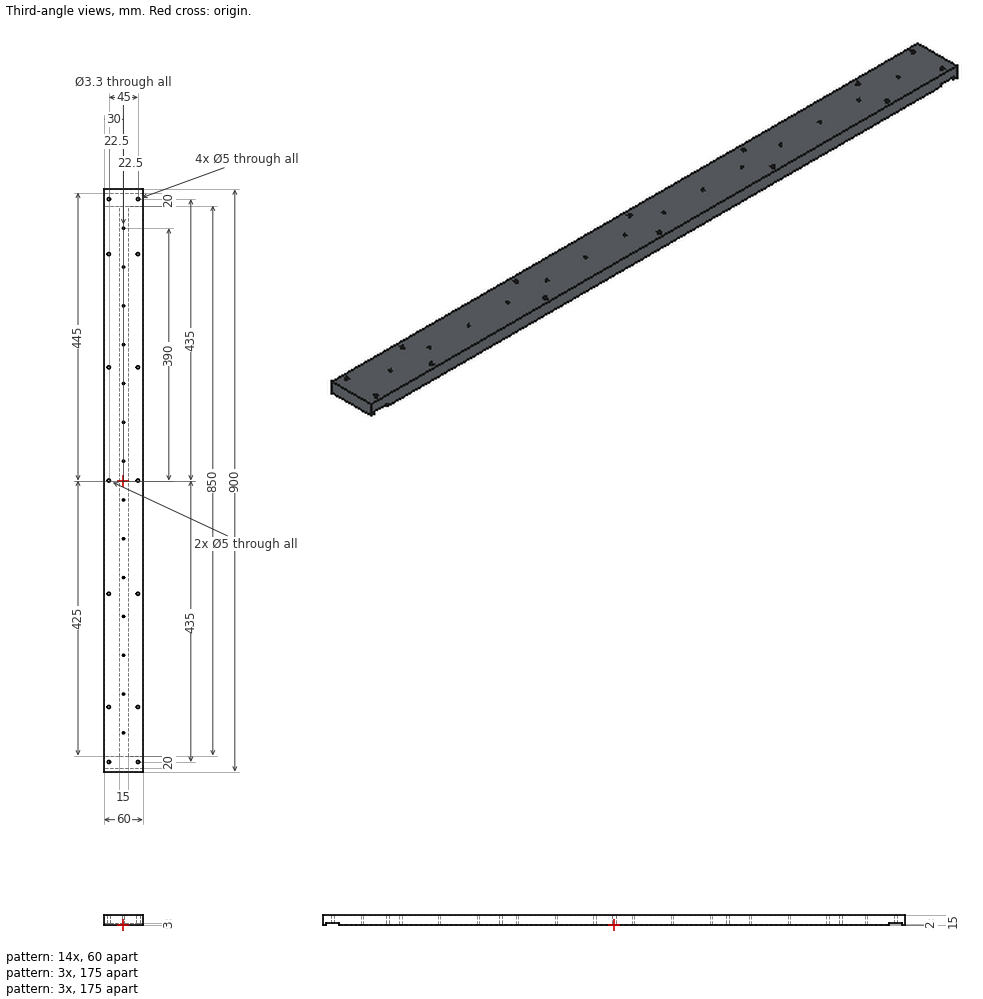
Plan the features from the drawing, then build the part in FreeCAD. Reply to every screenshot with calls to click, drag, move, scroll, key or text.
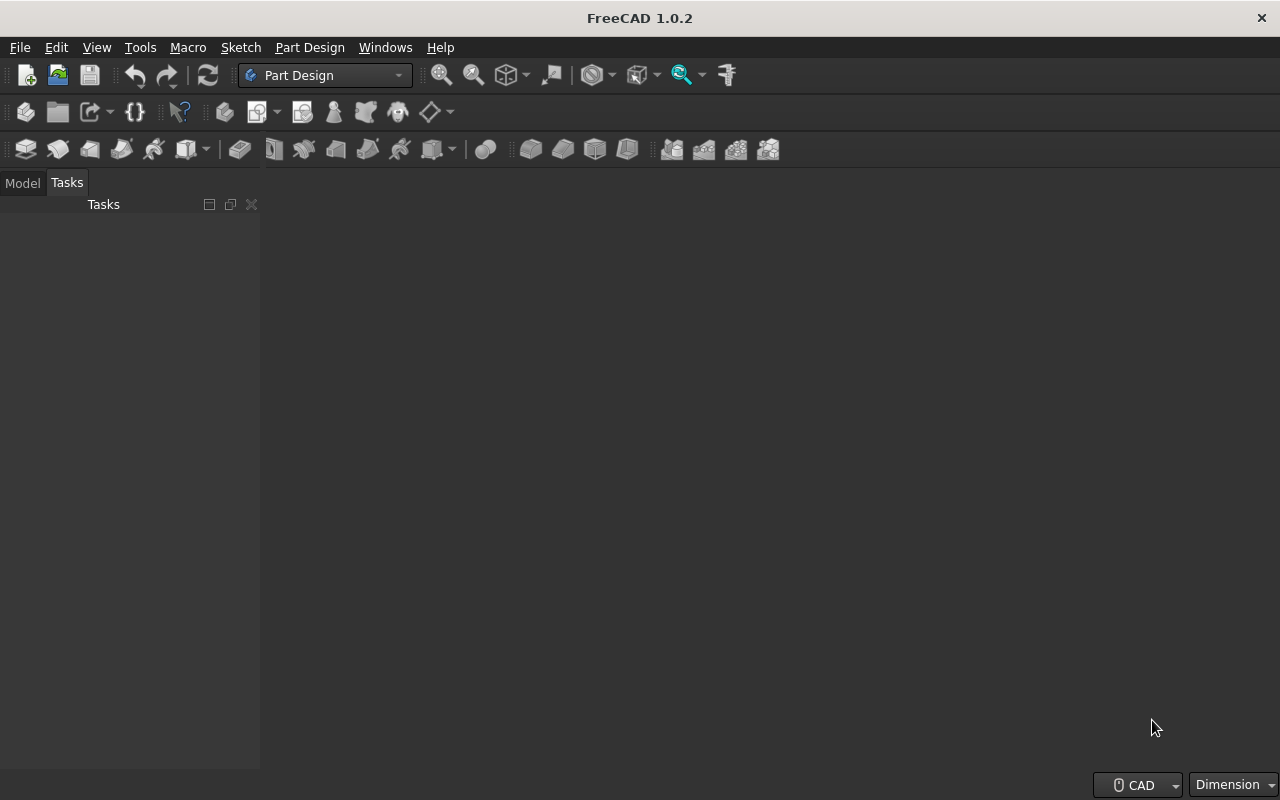
key(ctrl+n)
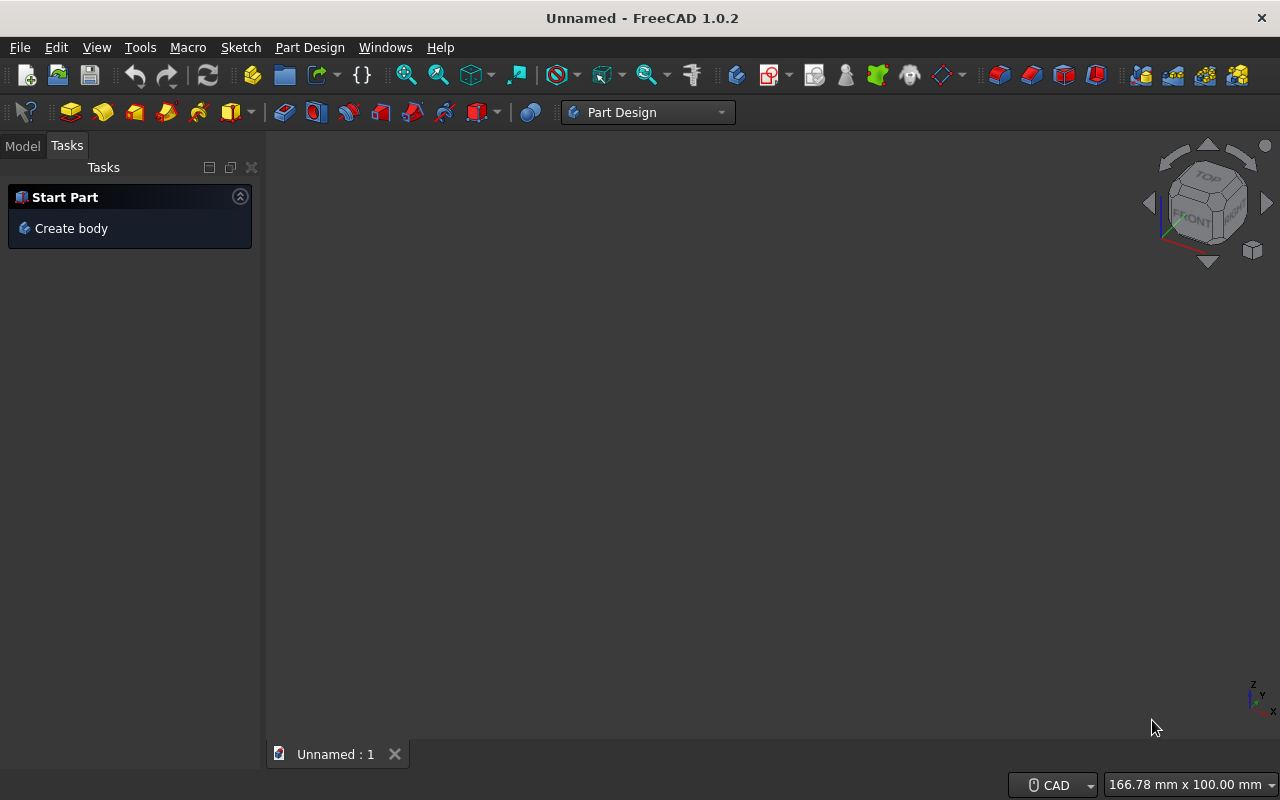
click(770, 76)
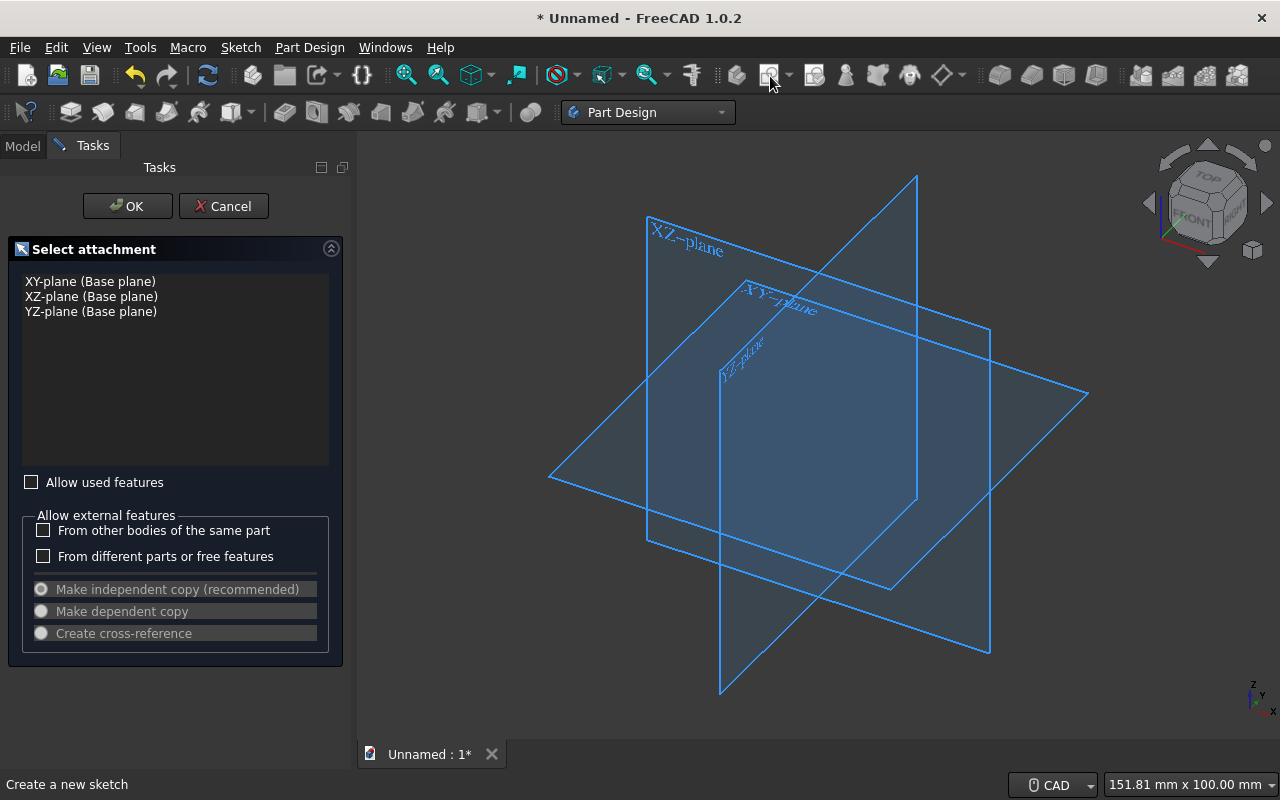
click(82, 282)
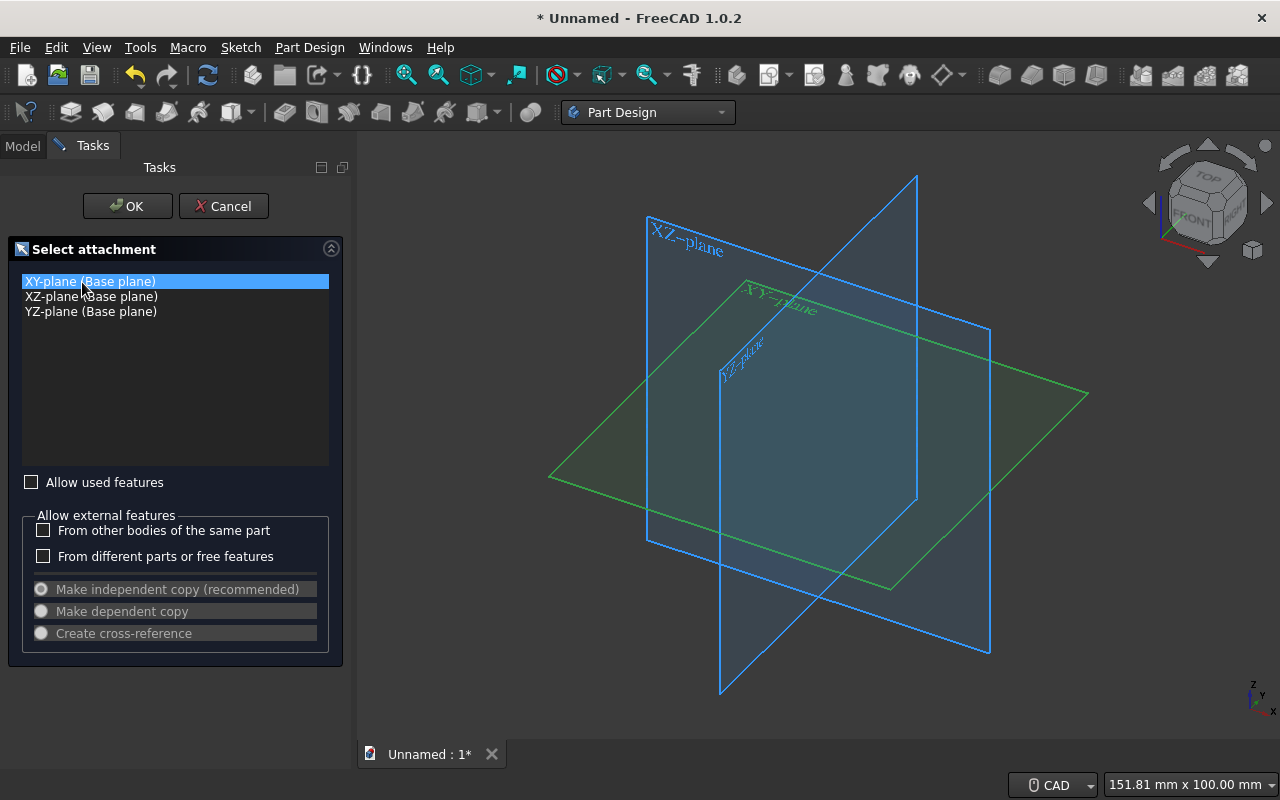
click(128, 206)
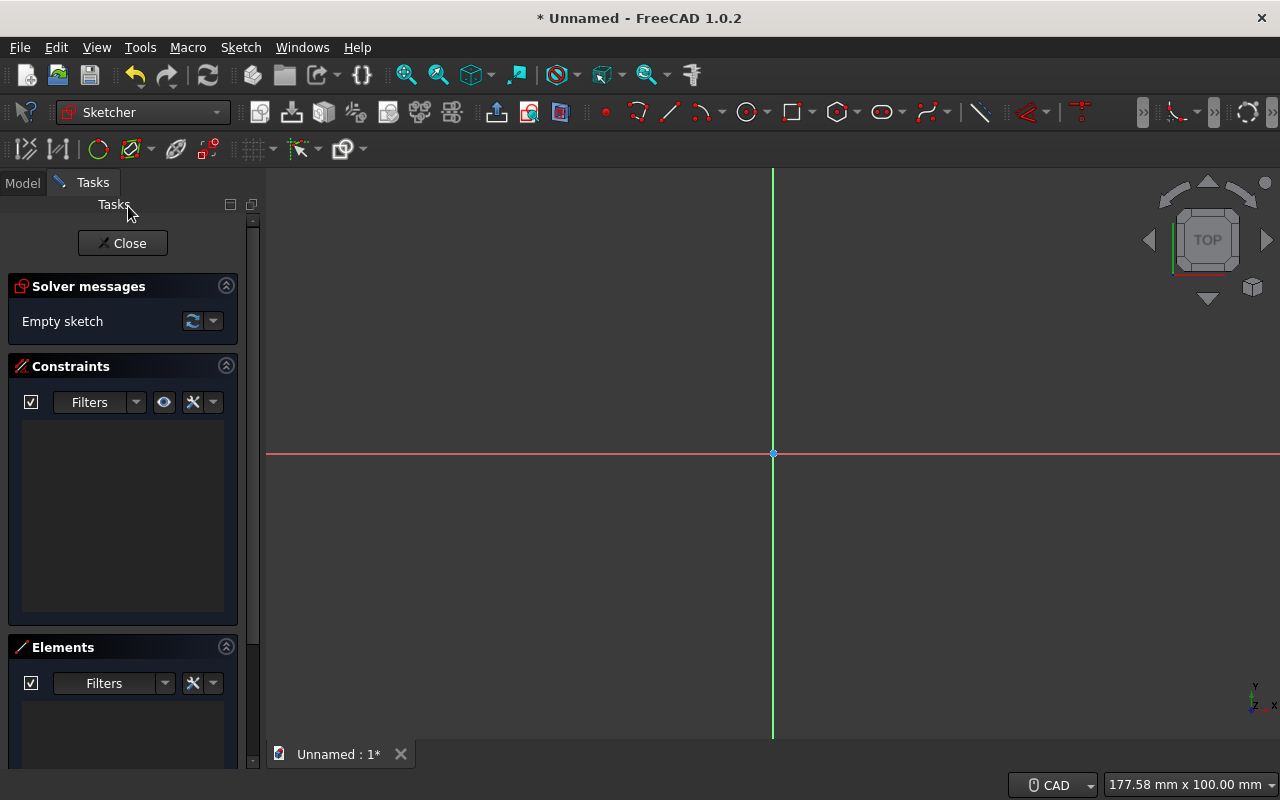
scroll(699, 454, down, 13)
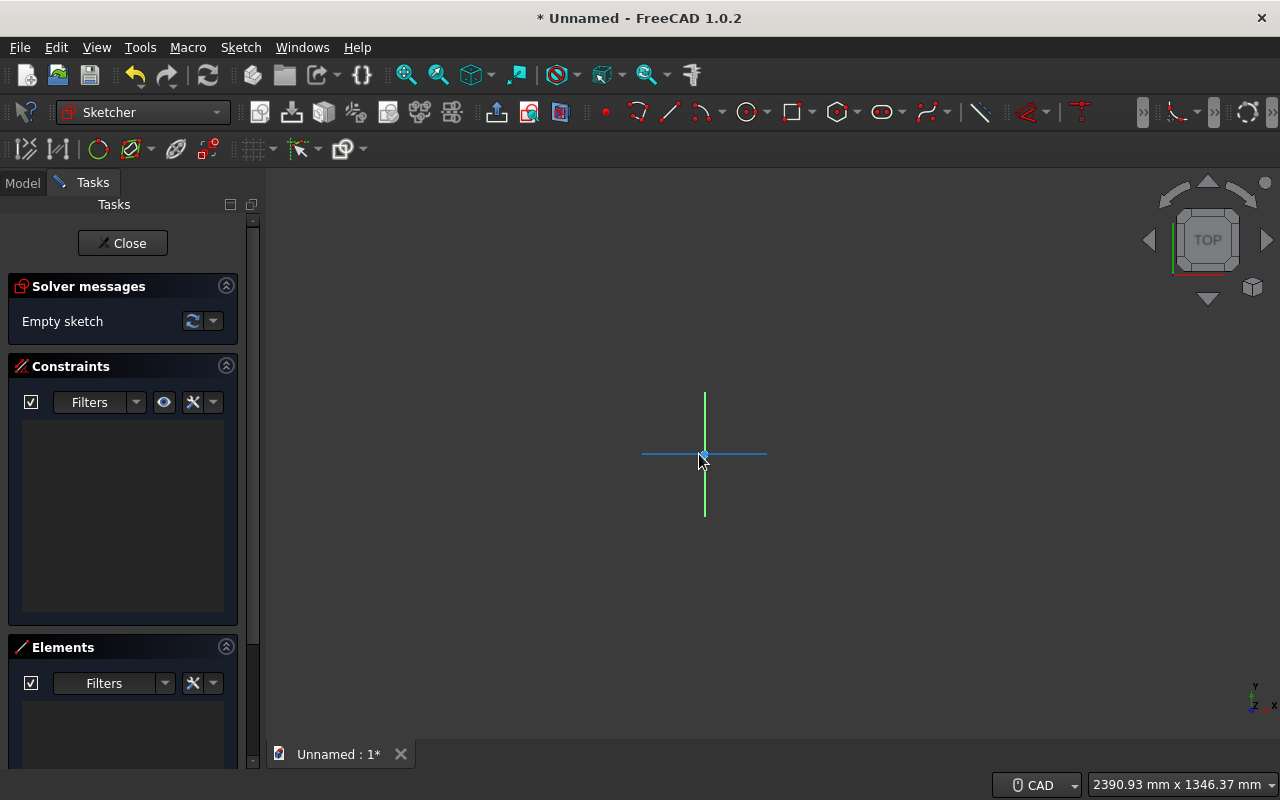
key(g)
key(v)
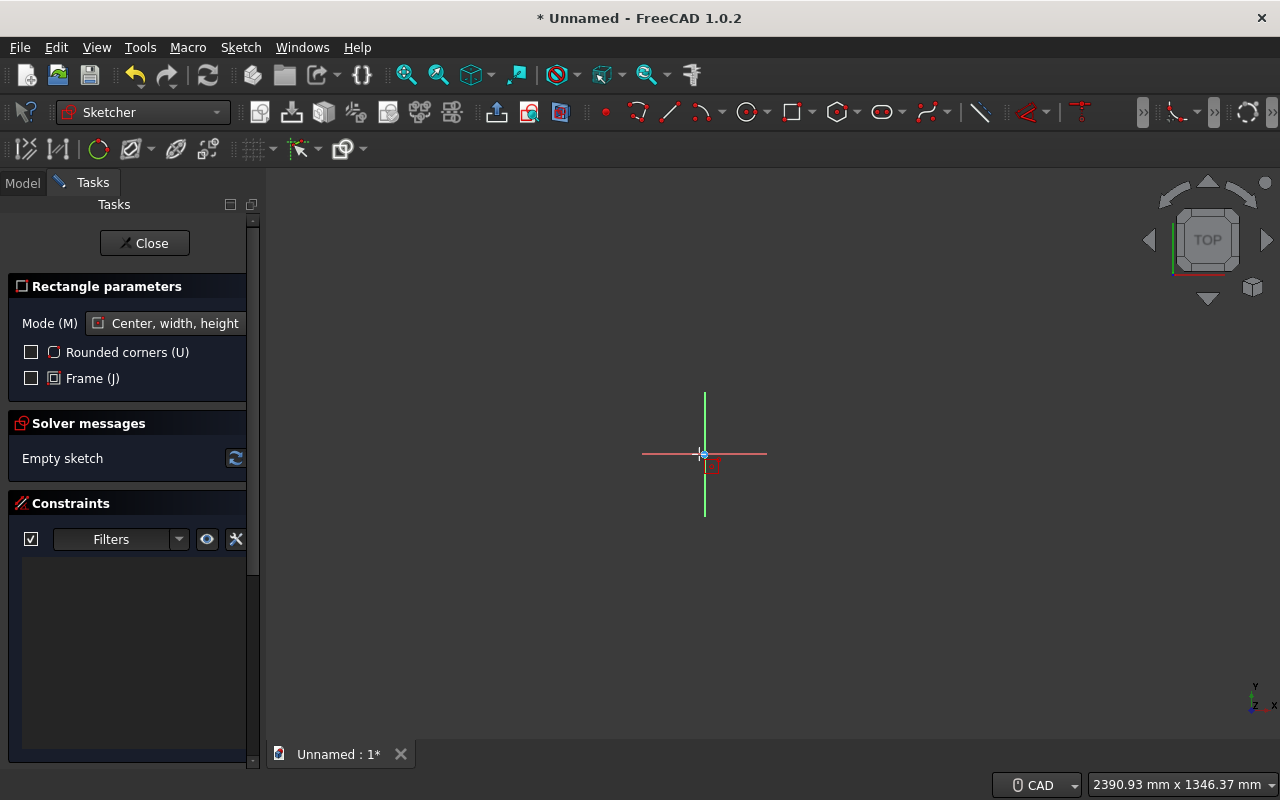
scroll(705, 454, up, 2)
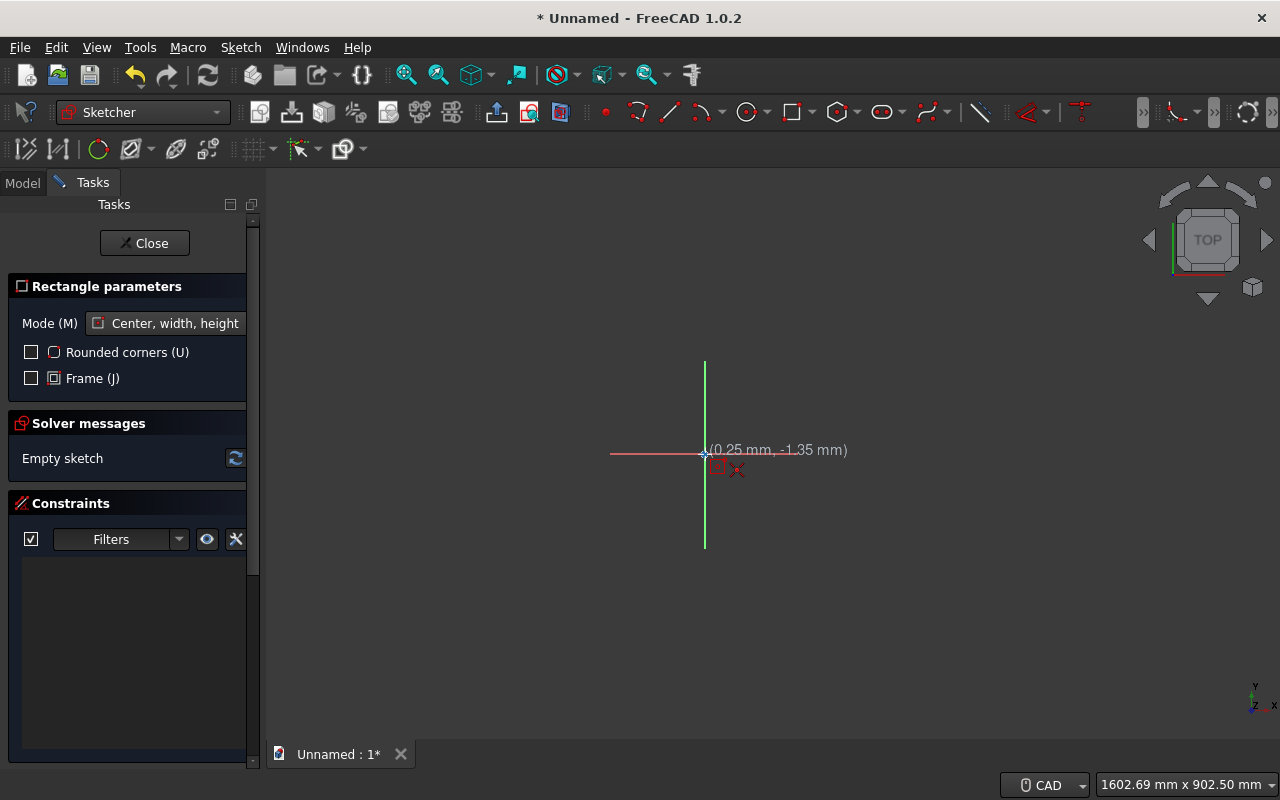
click(705, 454)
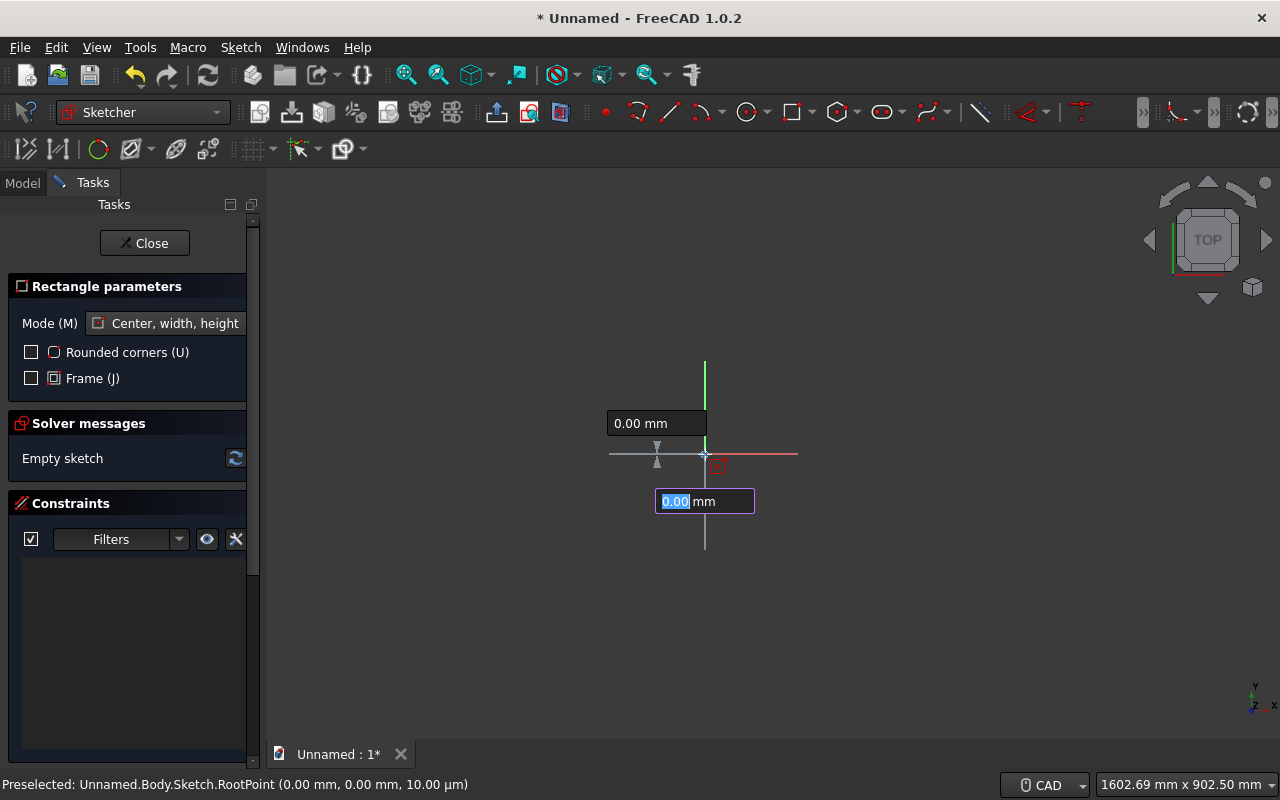
scroll(704, 452, down, 2)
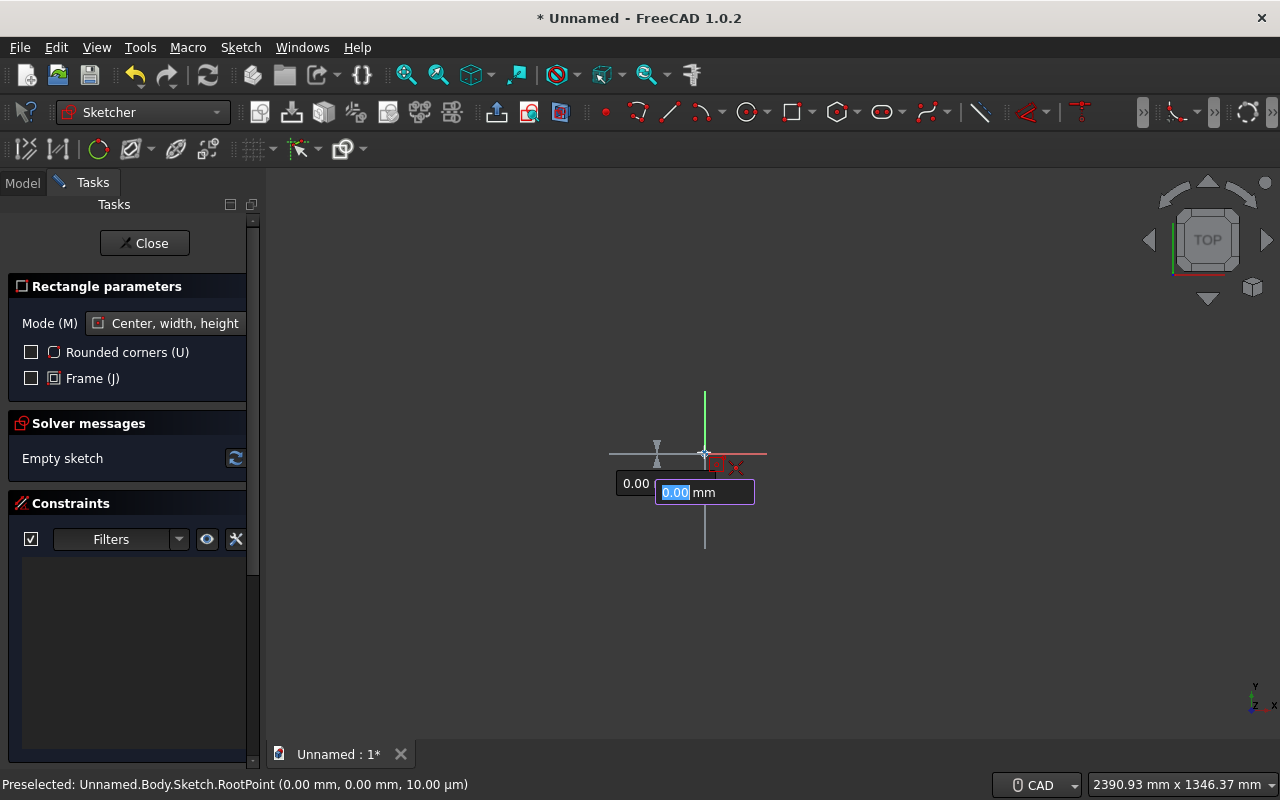
scroll(717, 263, up, 2)